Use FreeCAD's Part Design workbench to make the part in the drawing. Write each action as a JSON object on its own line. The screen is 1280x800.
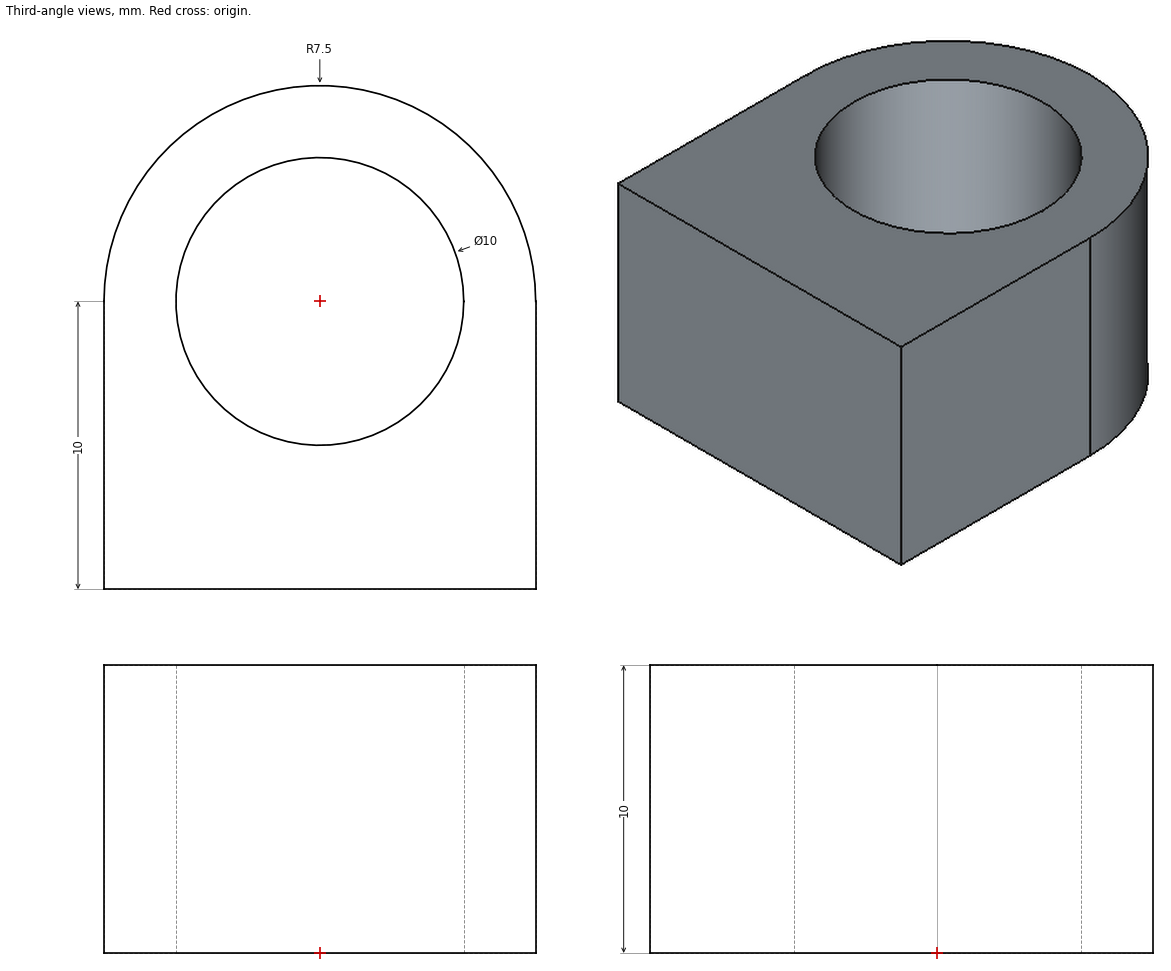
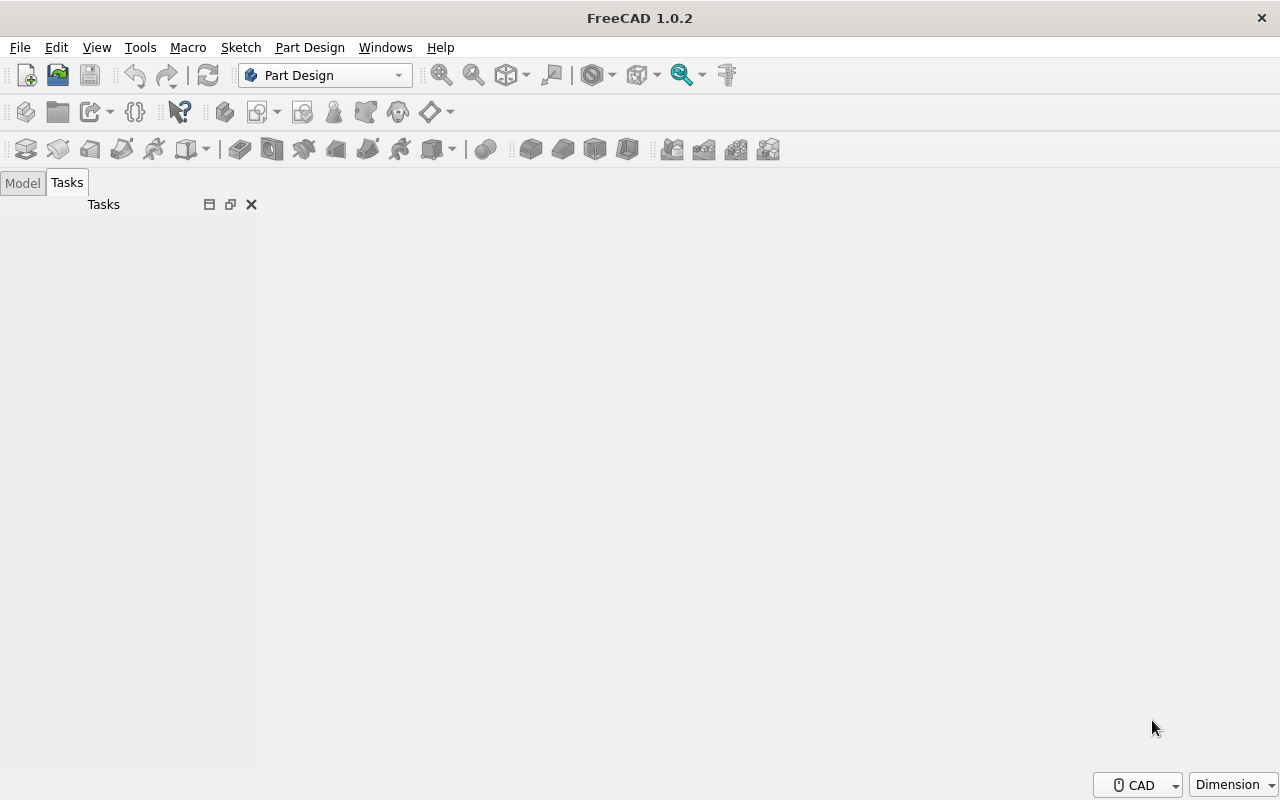
{"action": "left_click", "coordinate": [26, 76]}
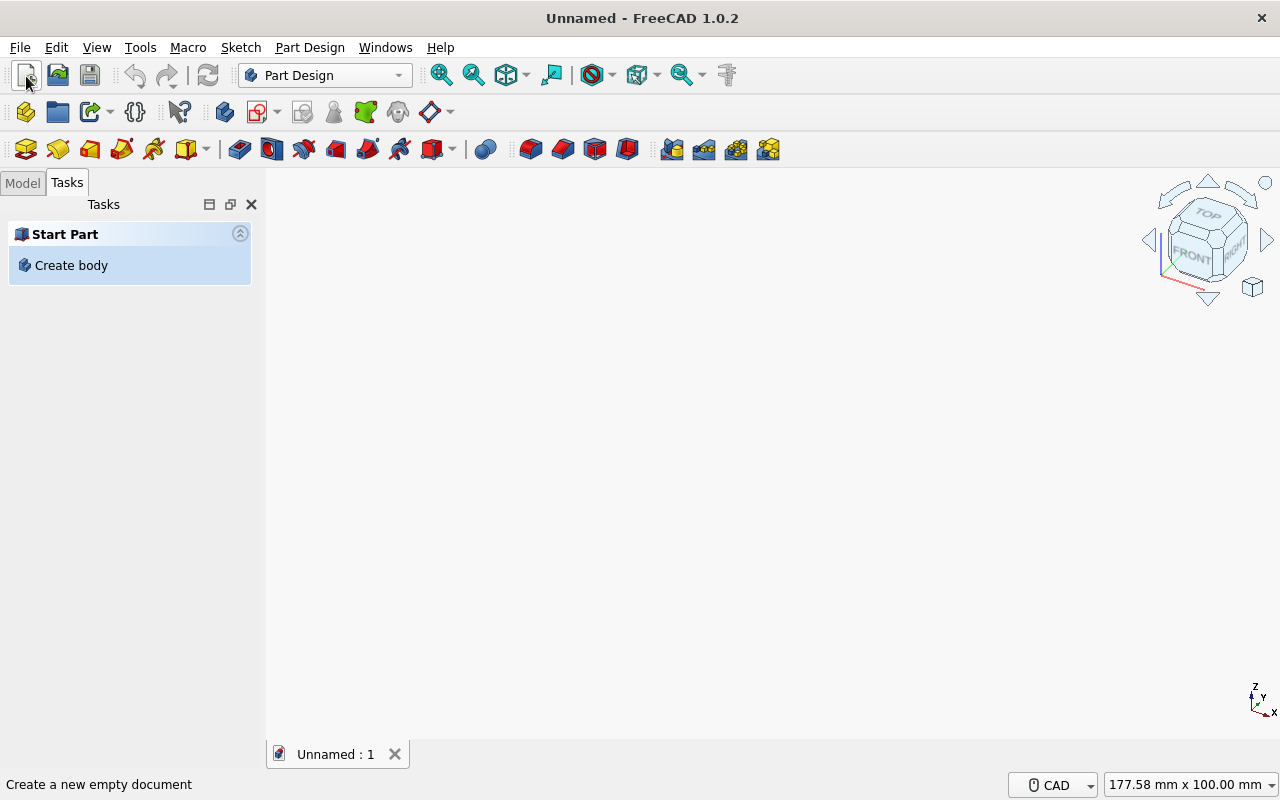
{"action": "left_click", "coordinate": [258, 112]}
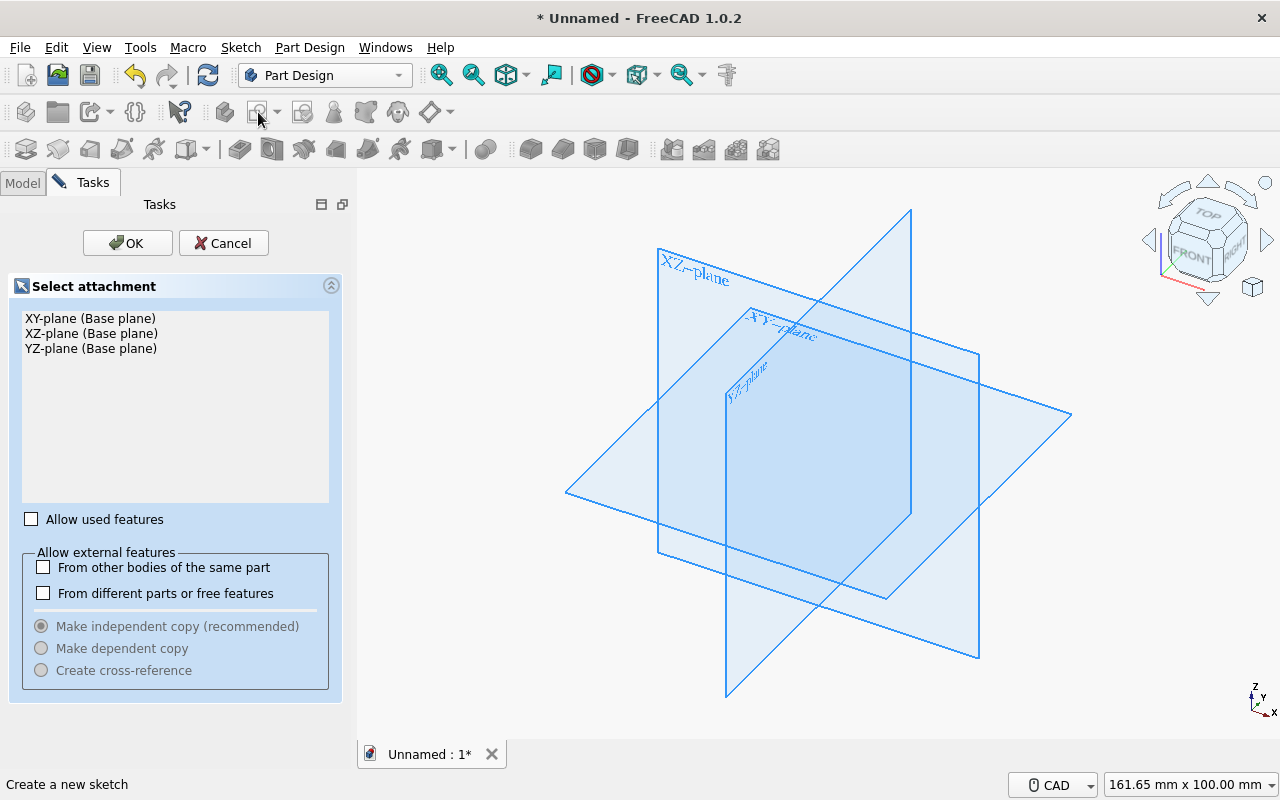
{"action": "left_click", "coordinate": [82, 318]}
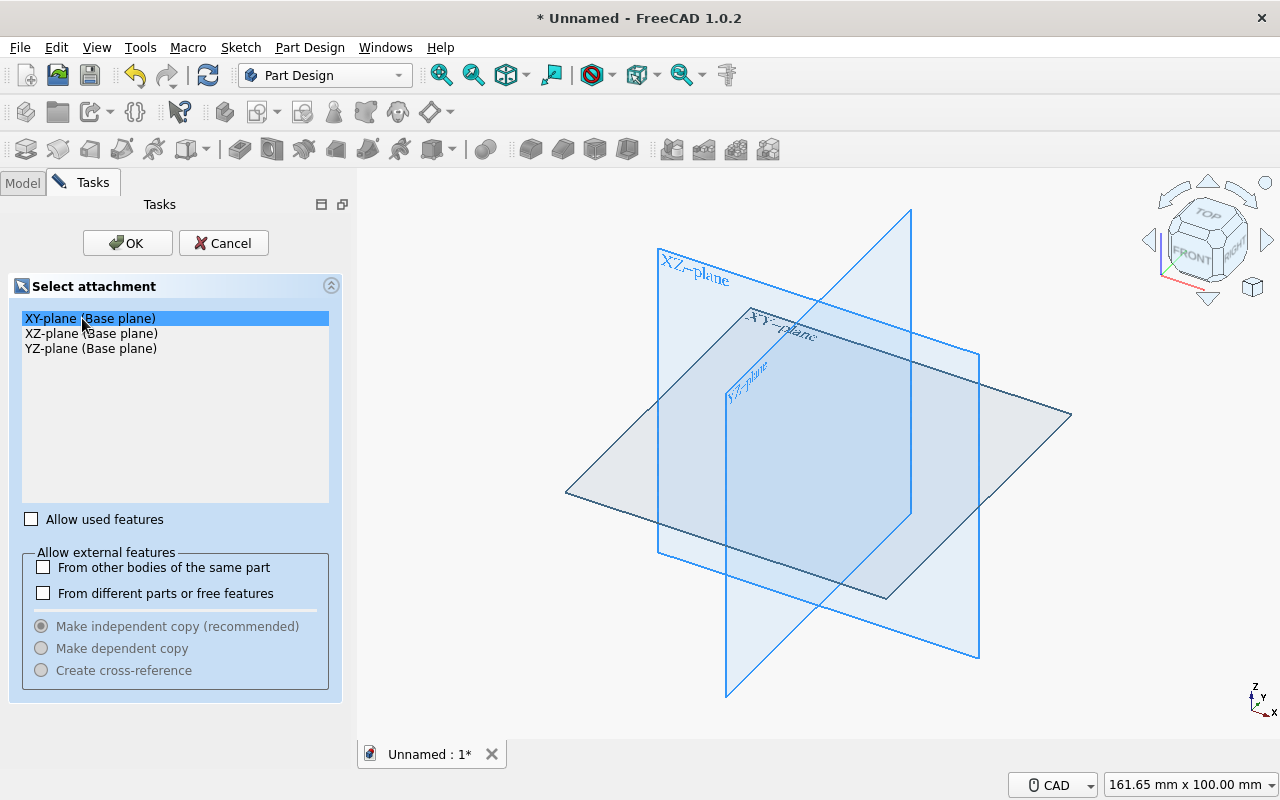
{"action": "left_click", "coordinate": [128, 243]}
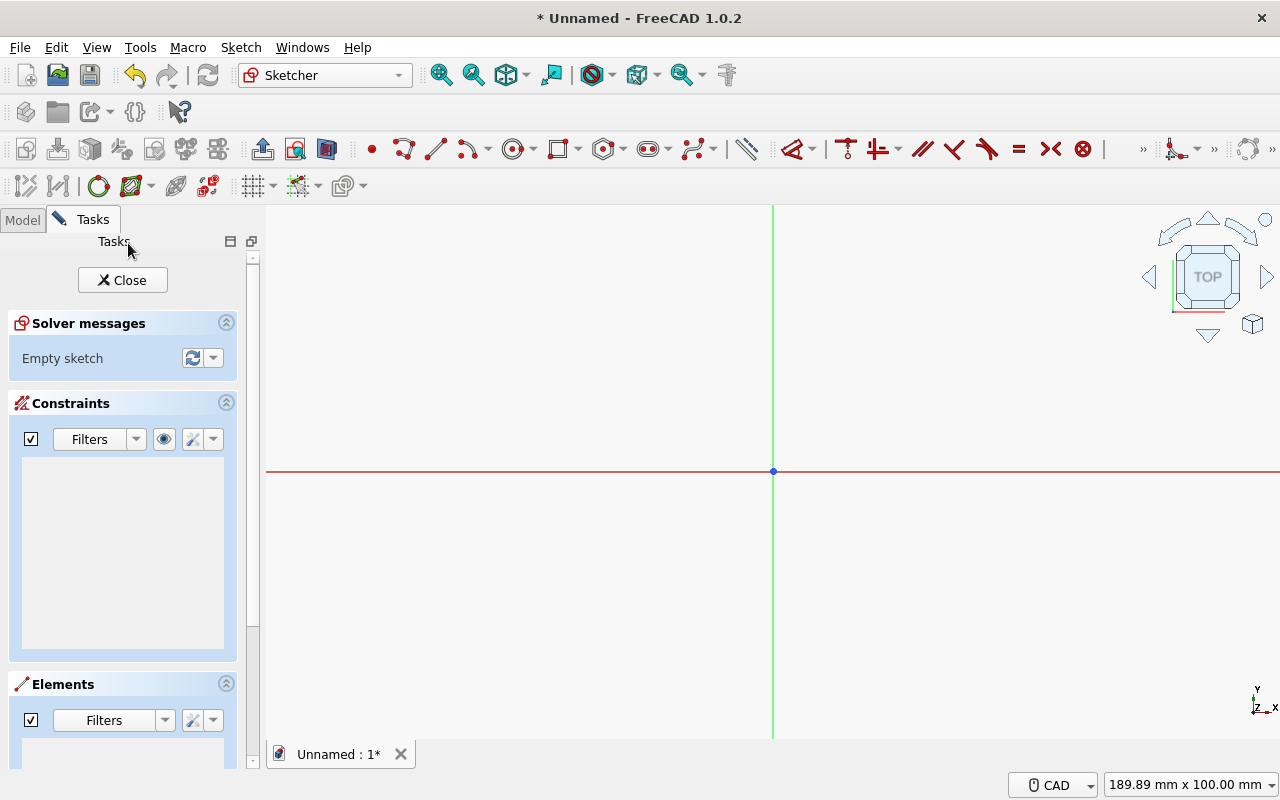
{"action": "scroll", "coordinate": [803, 482], "scroll_direction": "up", "scroll_amount": 6}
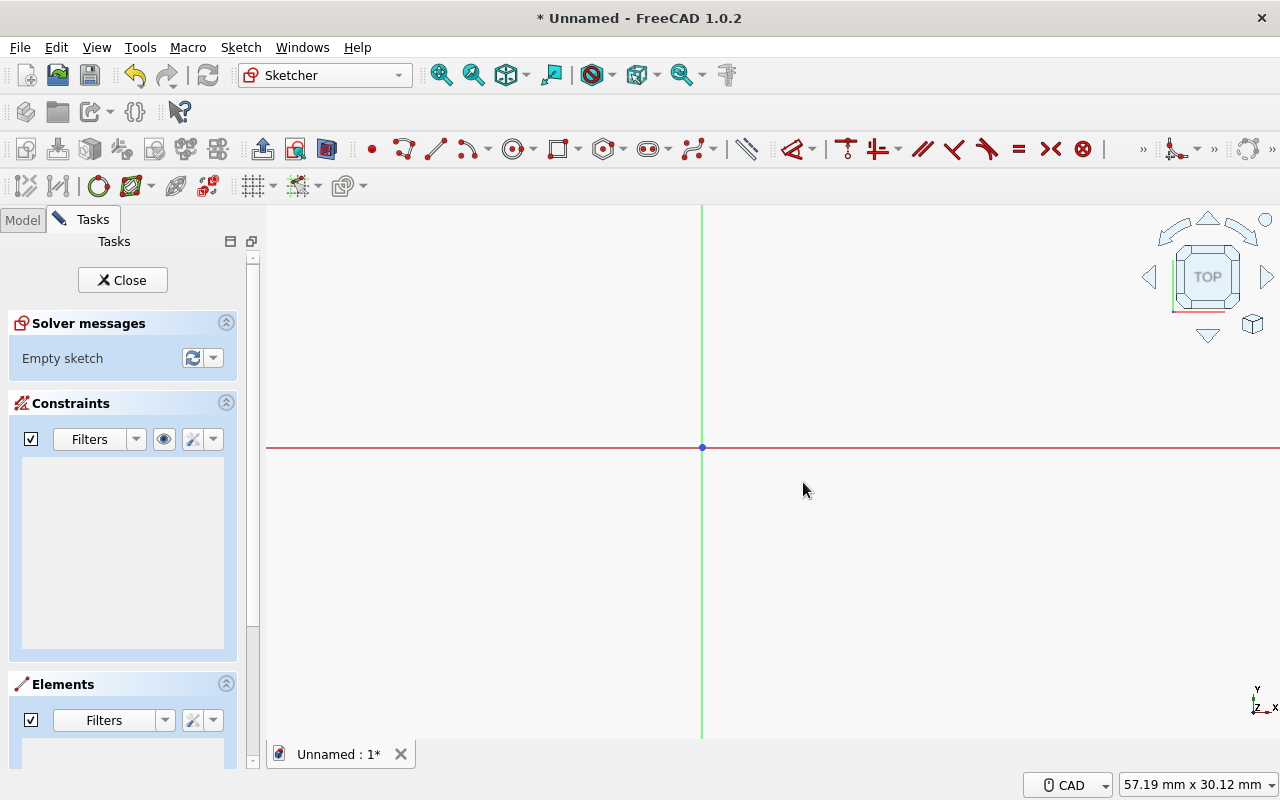
{"action": "left_click", "coordinate": [404, 150]}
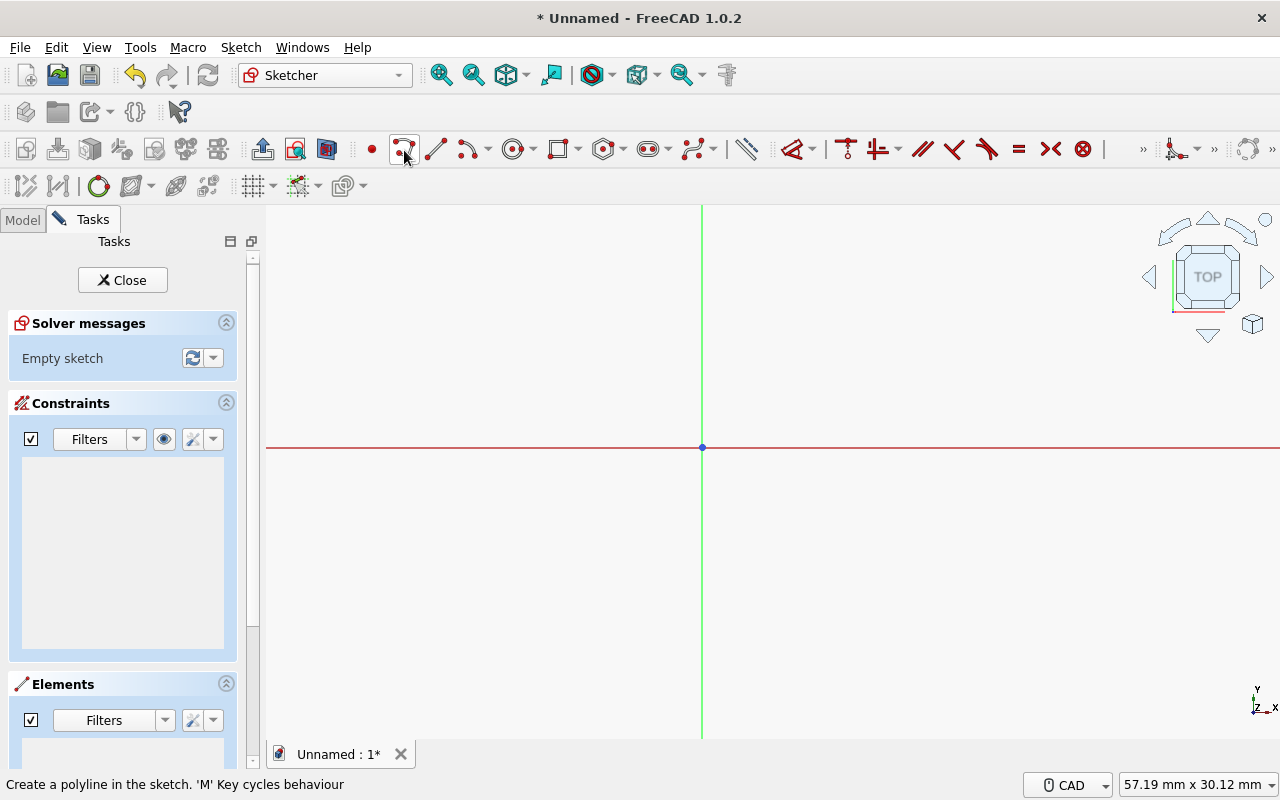
{"action": "left_click", "coordinate": [569, 448]}
{"action": "left_click", "coordinate": [569, 625]}
{"action": "left_click", "coordinate": [835, 625]}
{"action": "left_click", "coordinate": [835, 448]}
{"action": "right_click", "coordinate": [835, 448]}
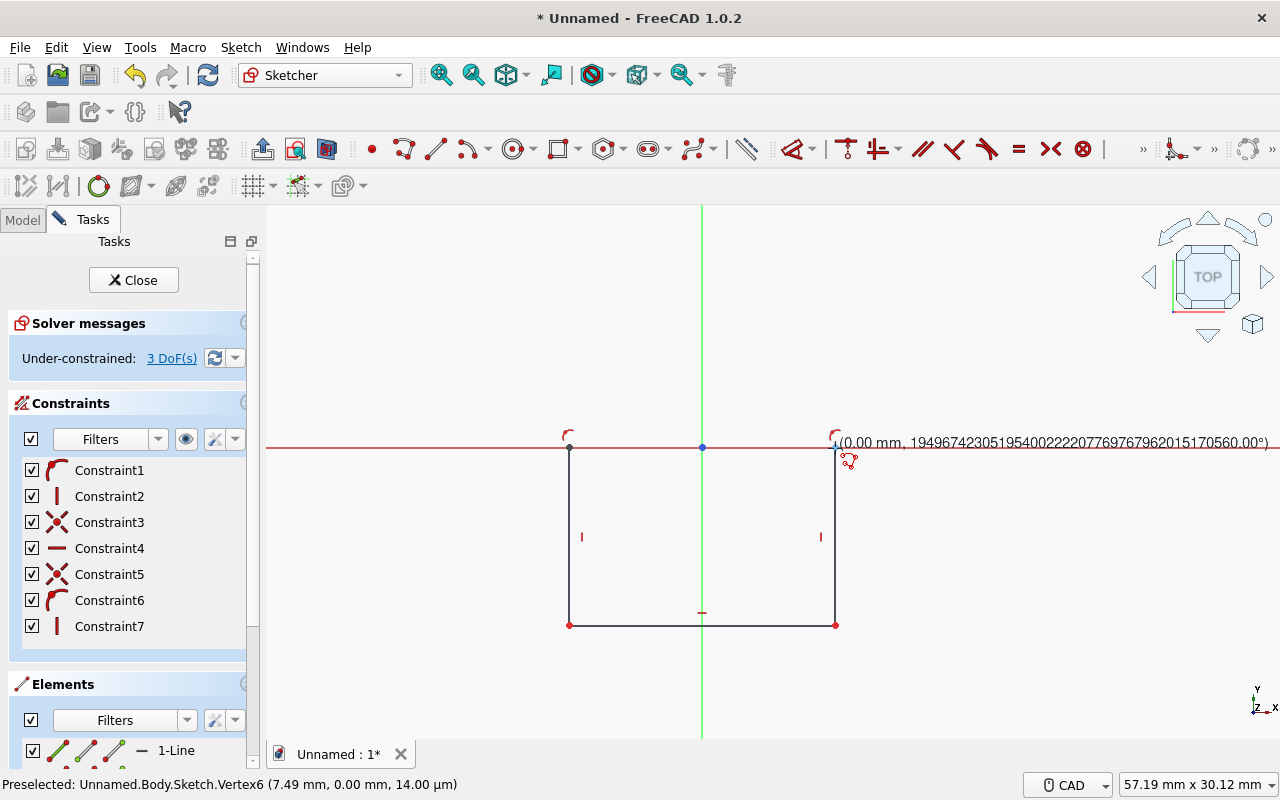
{"action": "key", "text": "g 3 a"}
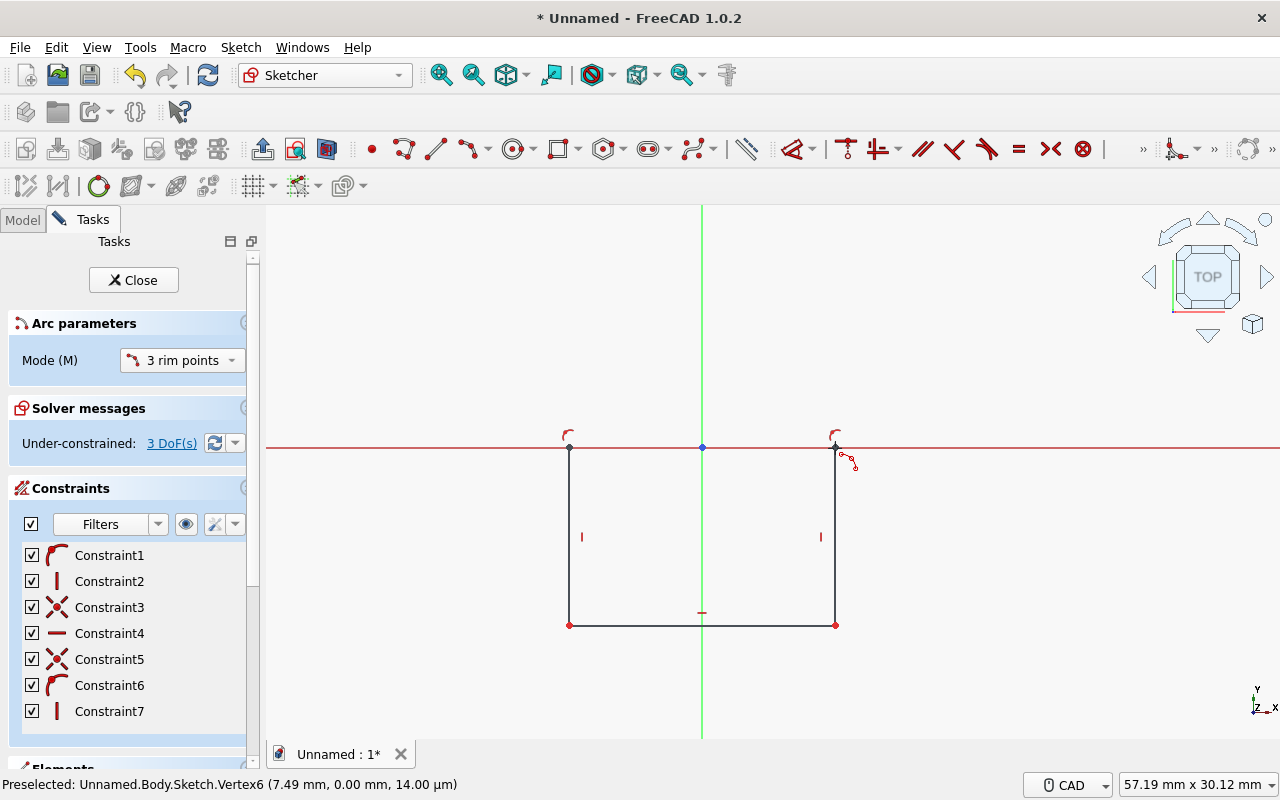
{"action": "left_click", "coordinate": [835, 448]}
{"action": "left_click", "coordinate": [569, 448]}
{"action": "left_click", "coordinate": [743, 321]}